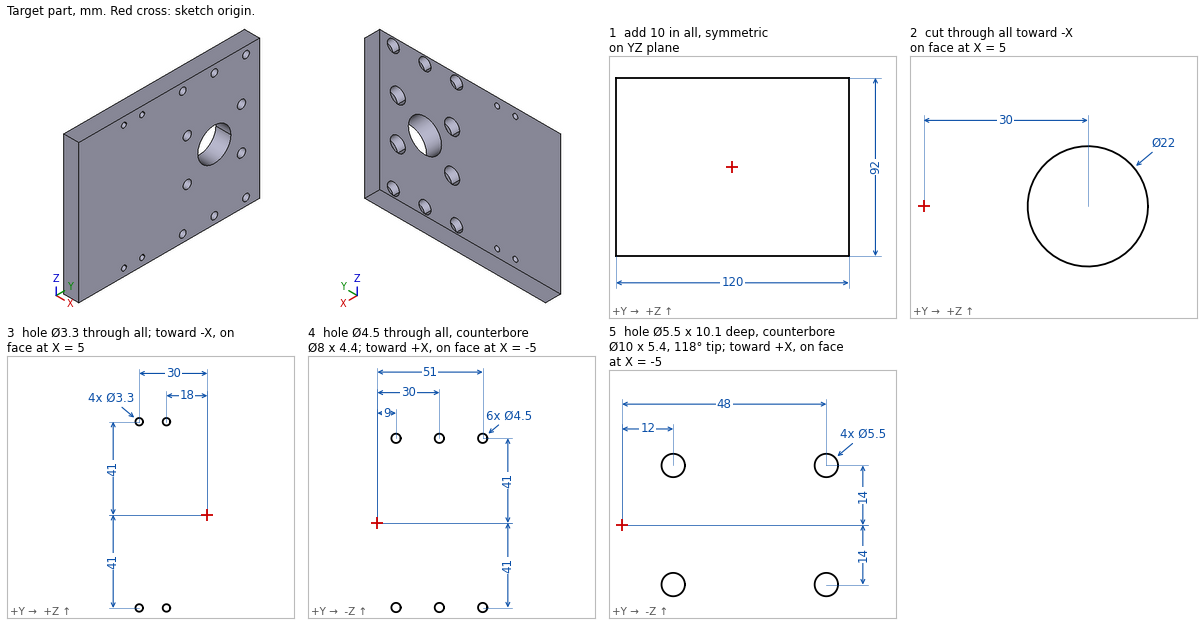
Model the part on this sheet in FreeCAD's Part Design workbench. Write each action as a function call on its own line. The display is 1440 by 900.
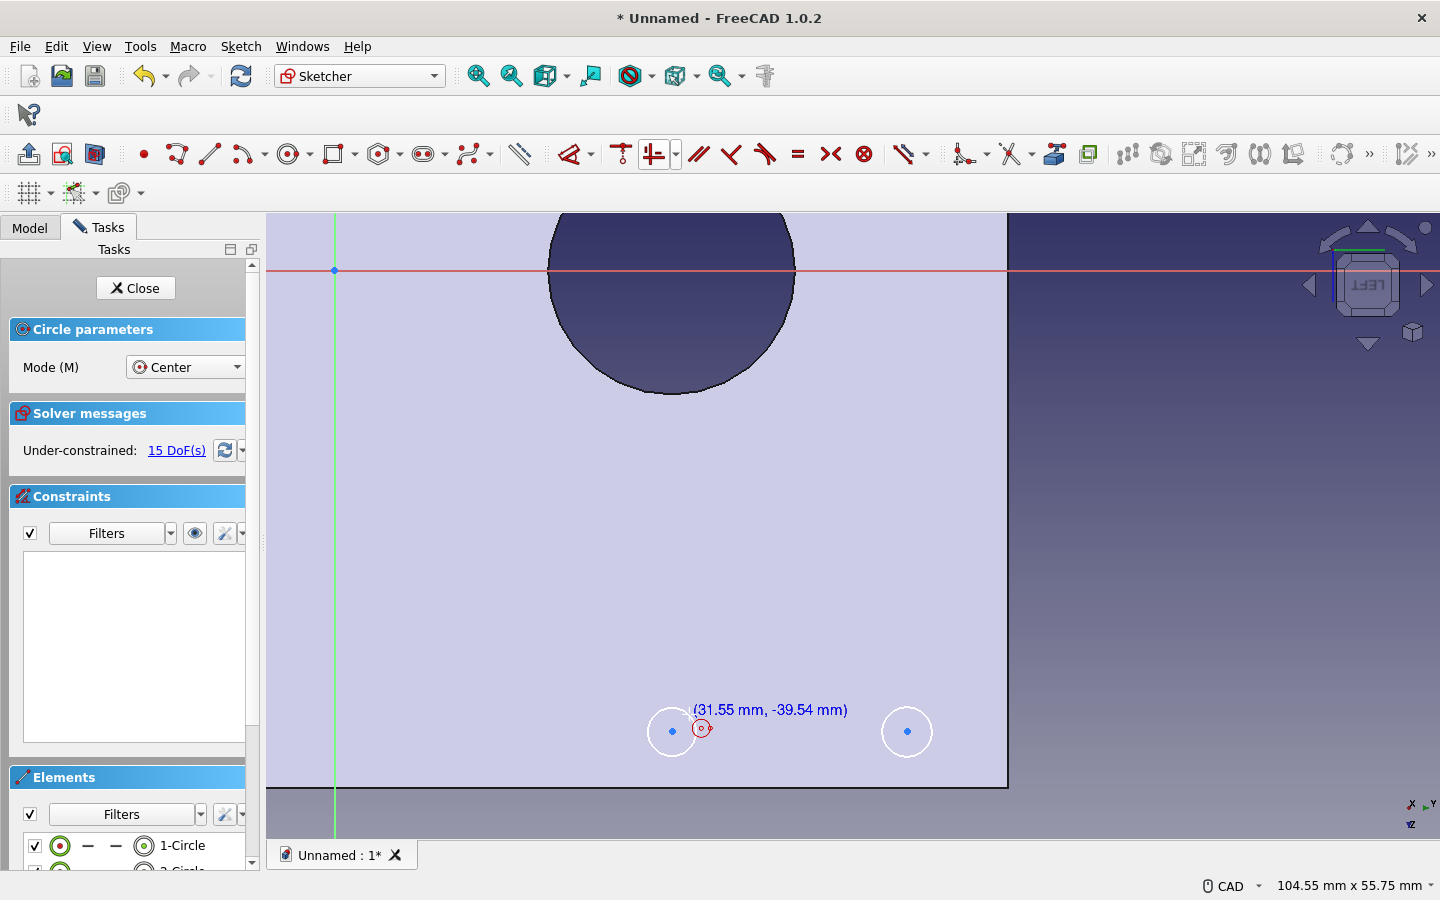
click(436, 731)
click(454, 714)
key(Escape)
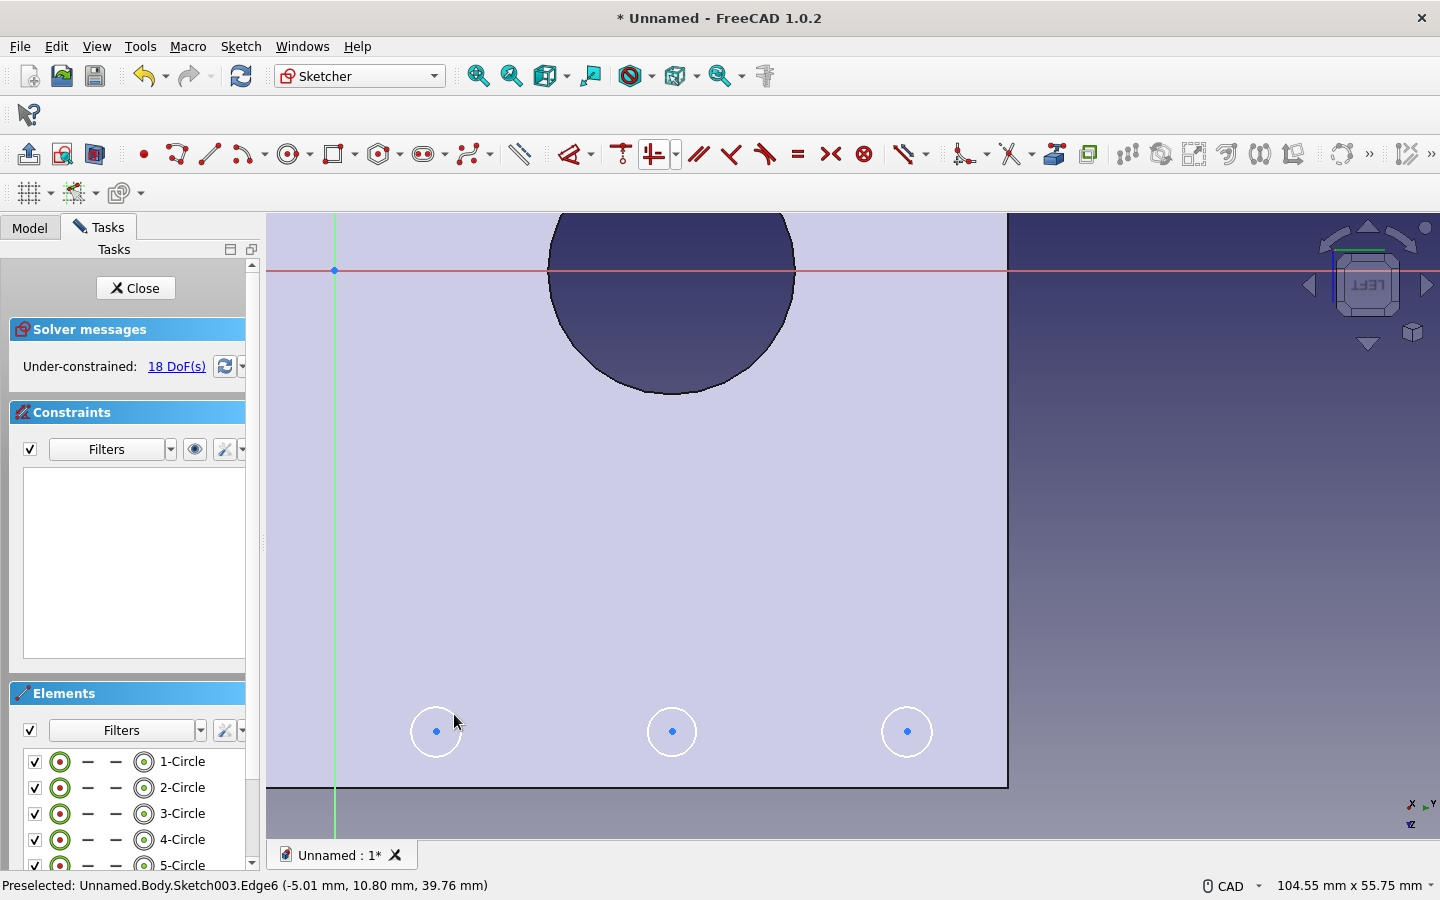
scroll(908, 734, down, 4)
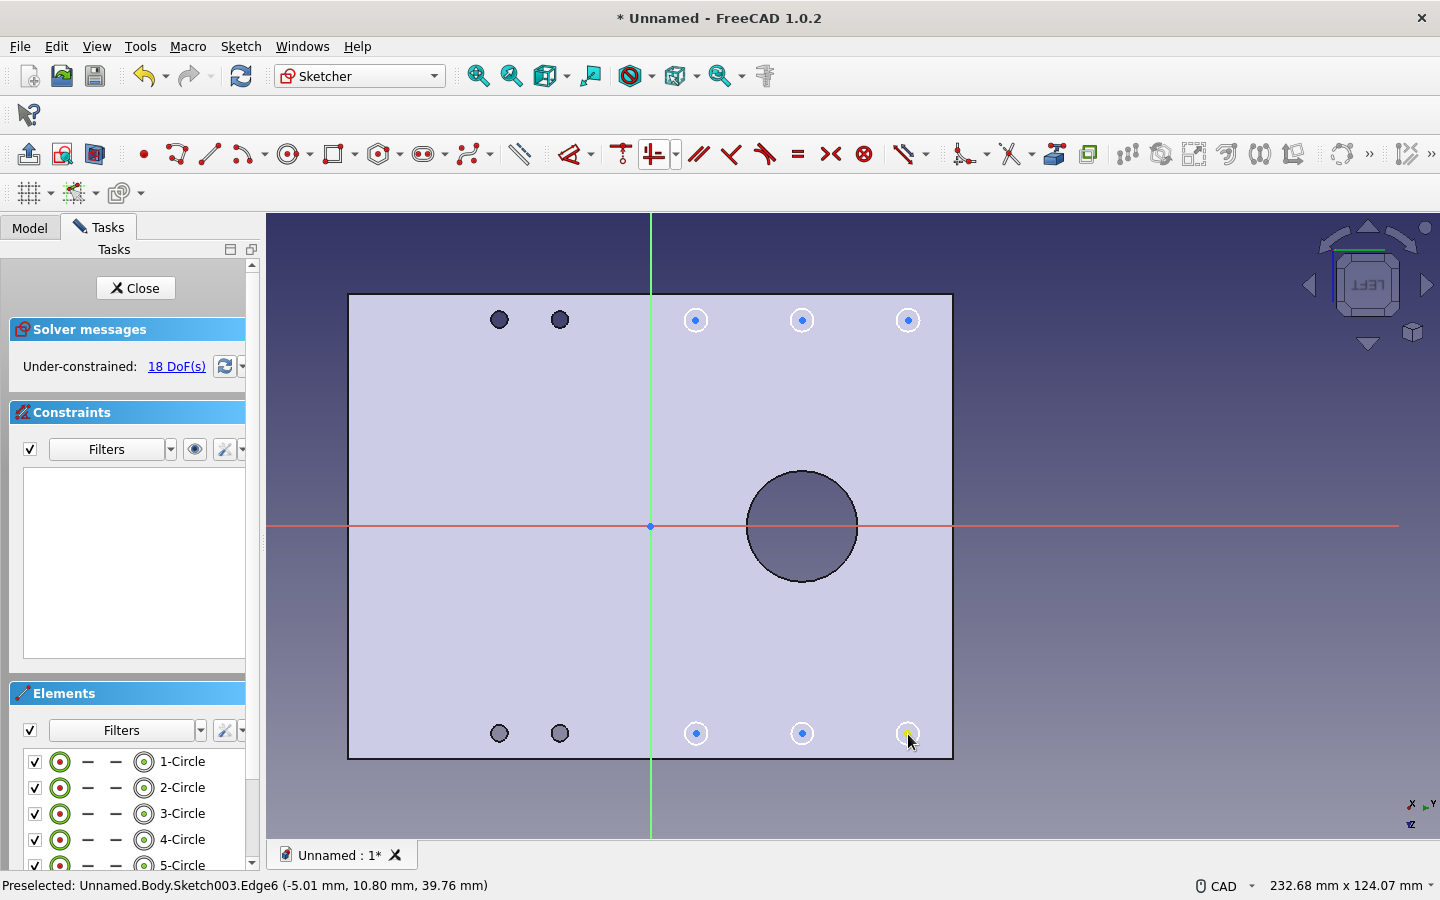
click(916, 312)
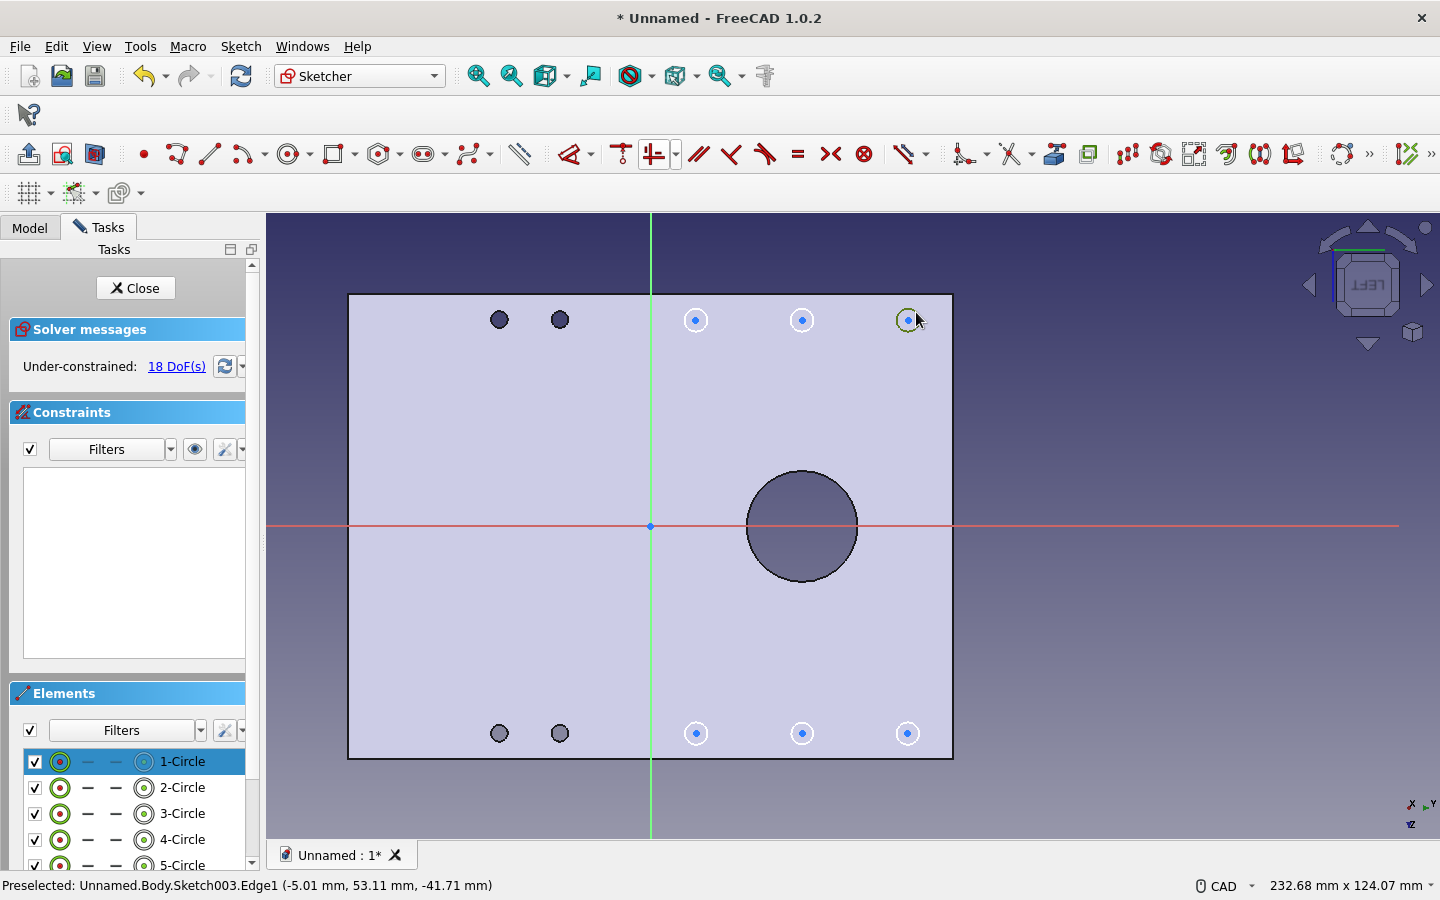
click(810, 312)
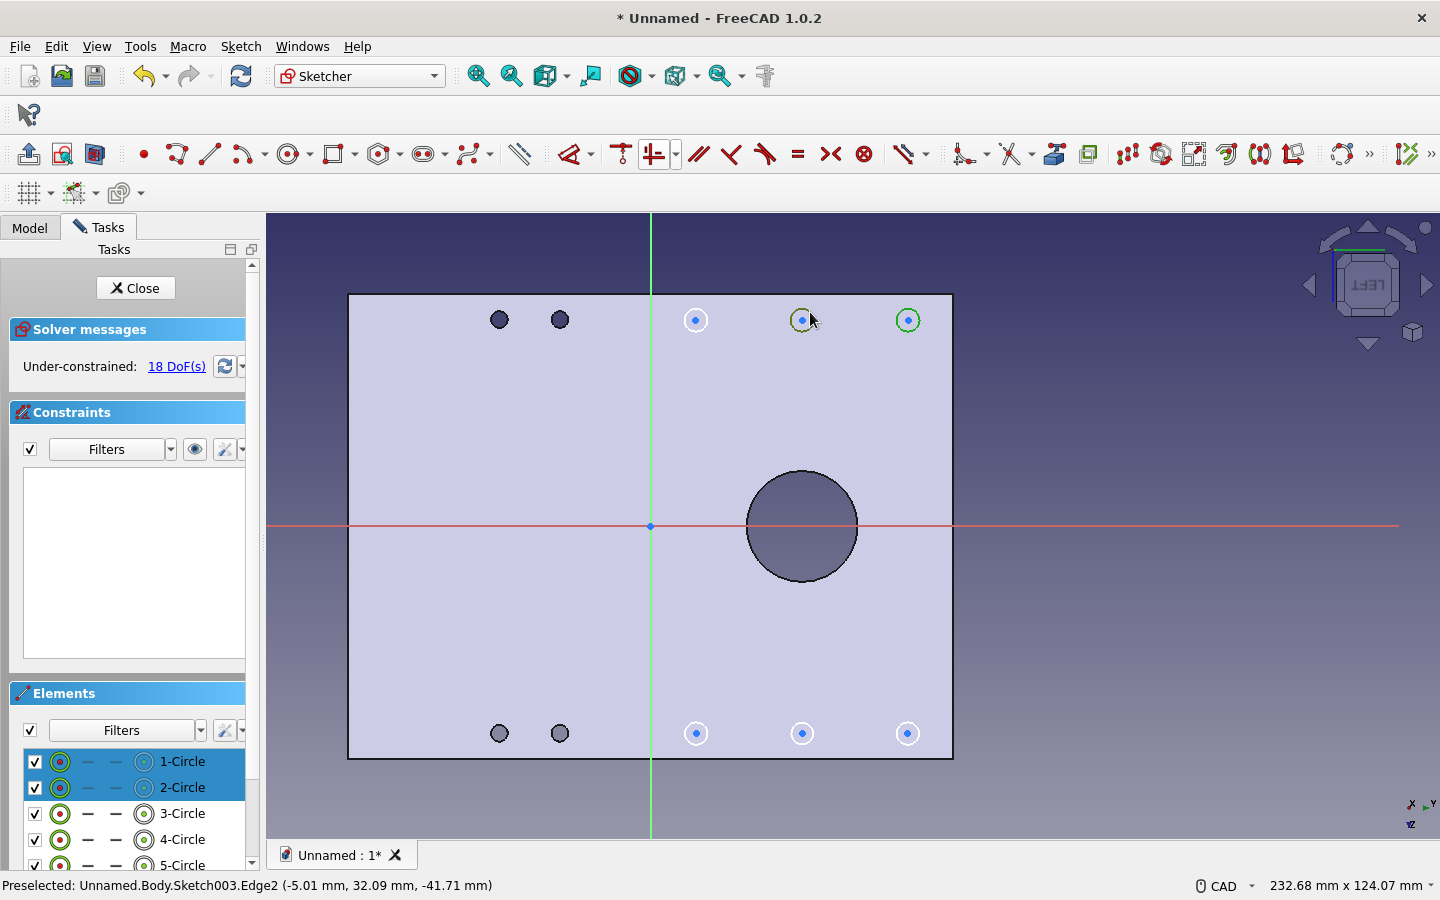
click(704, 312)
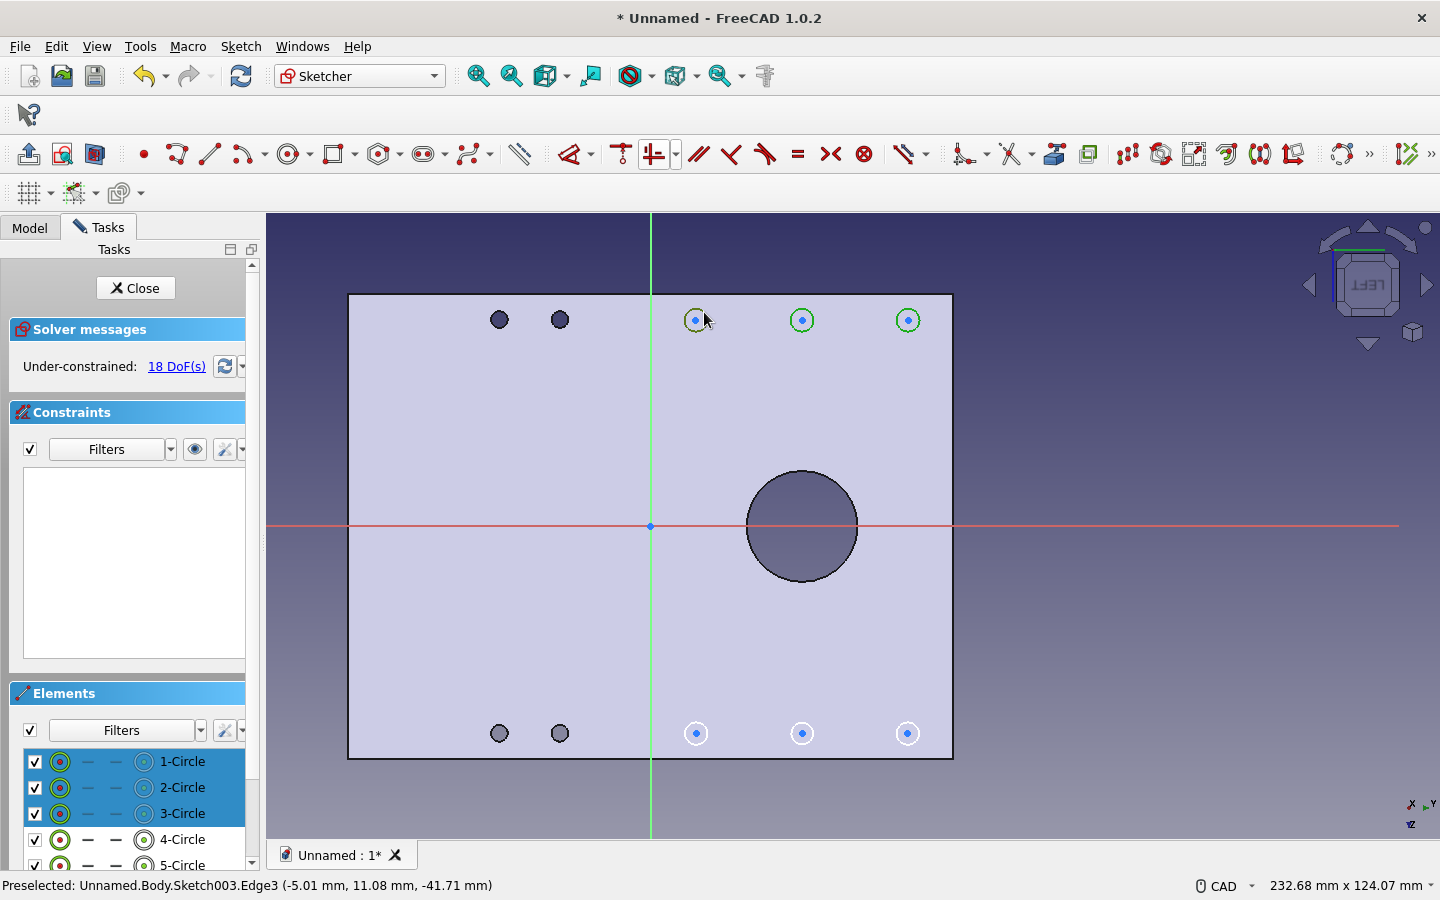
scroll(916, 726, up, 2)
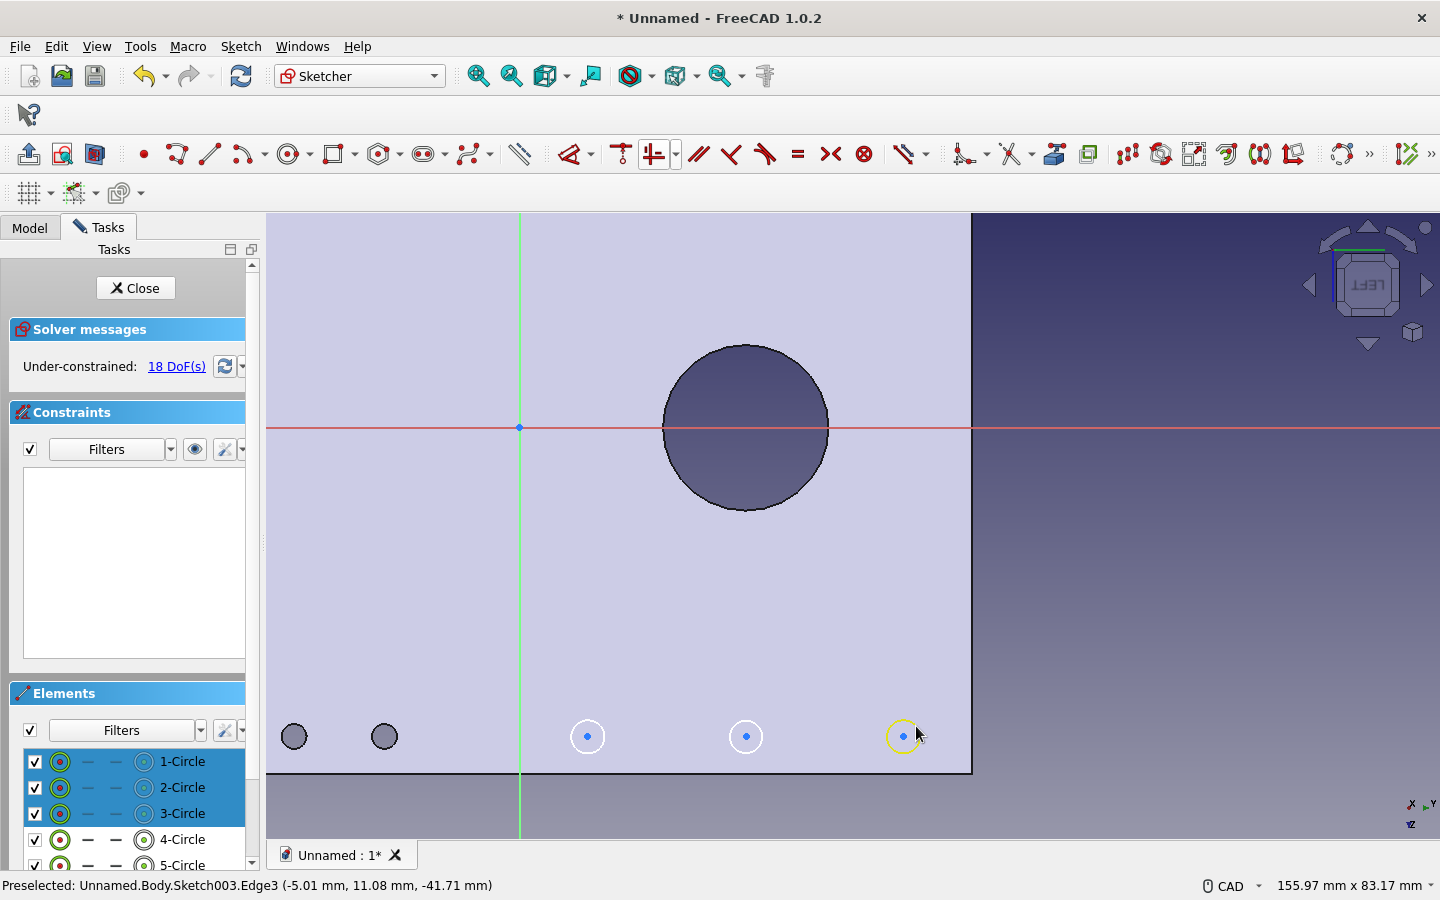
click(915, 725)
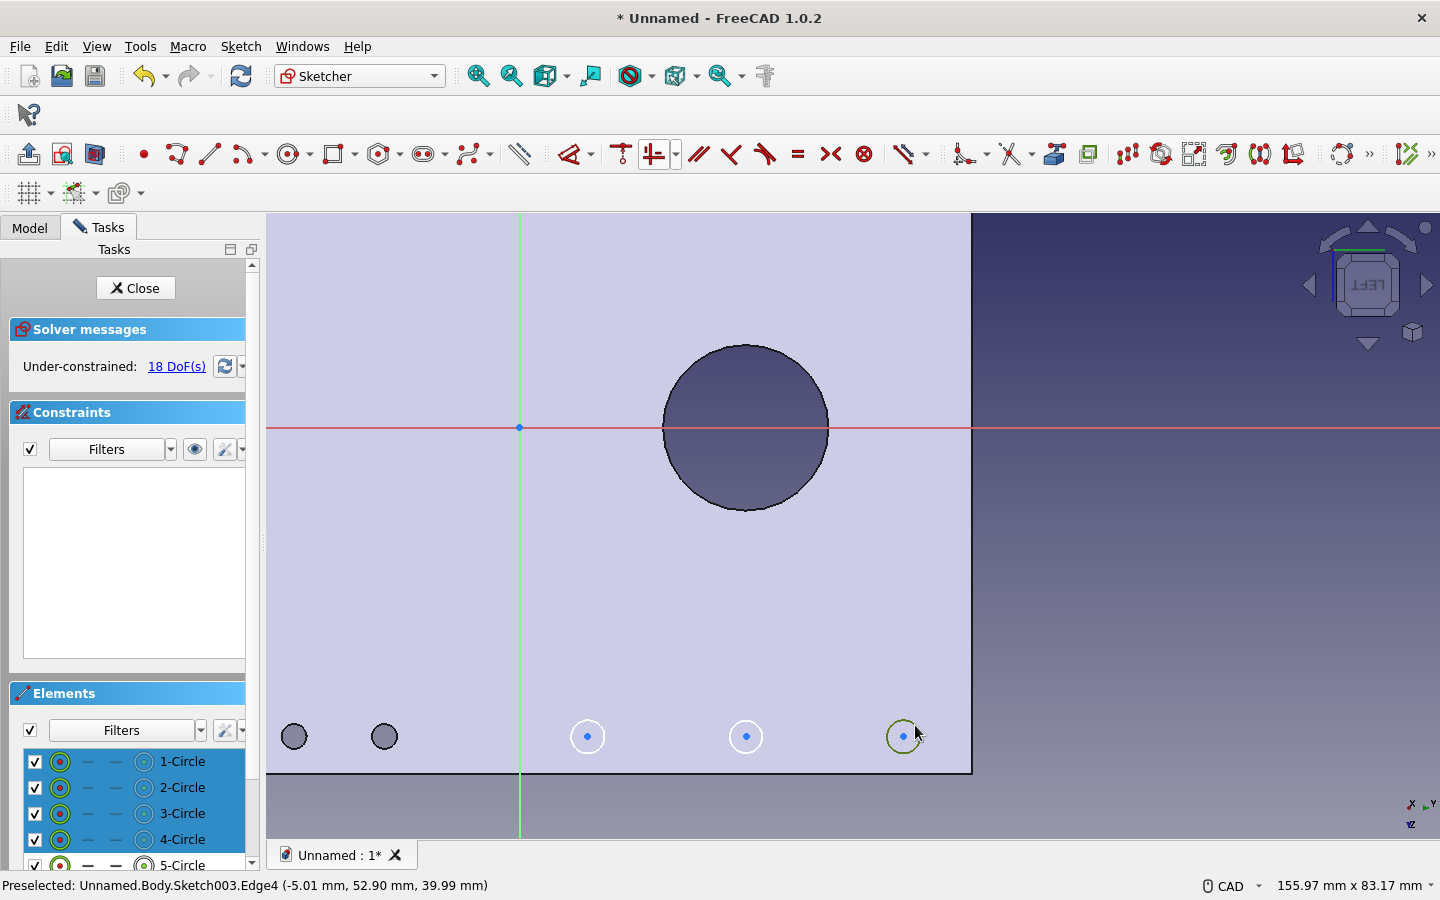
click(757, 725)